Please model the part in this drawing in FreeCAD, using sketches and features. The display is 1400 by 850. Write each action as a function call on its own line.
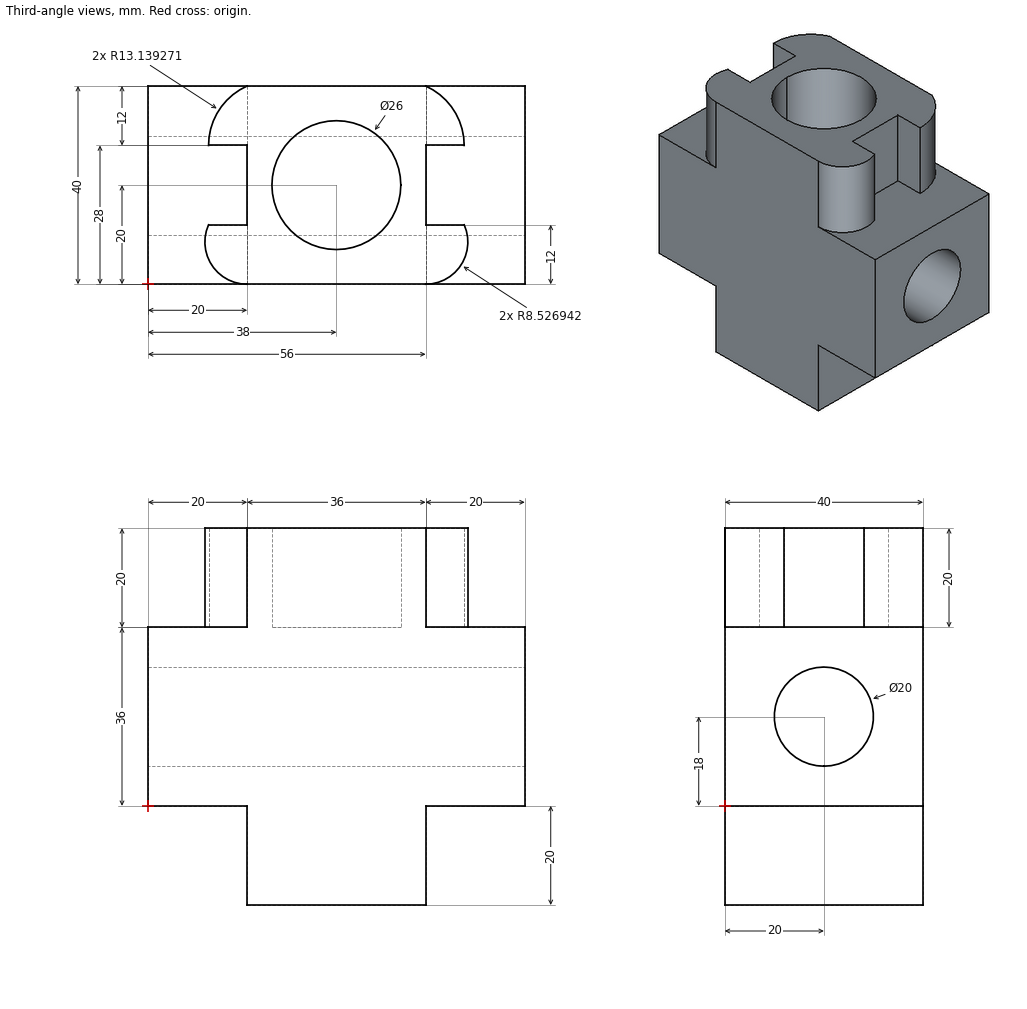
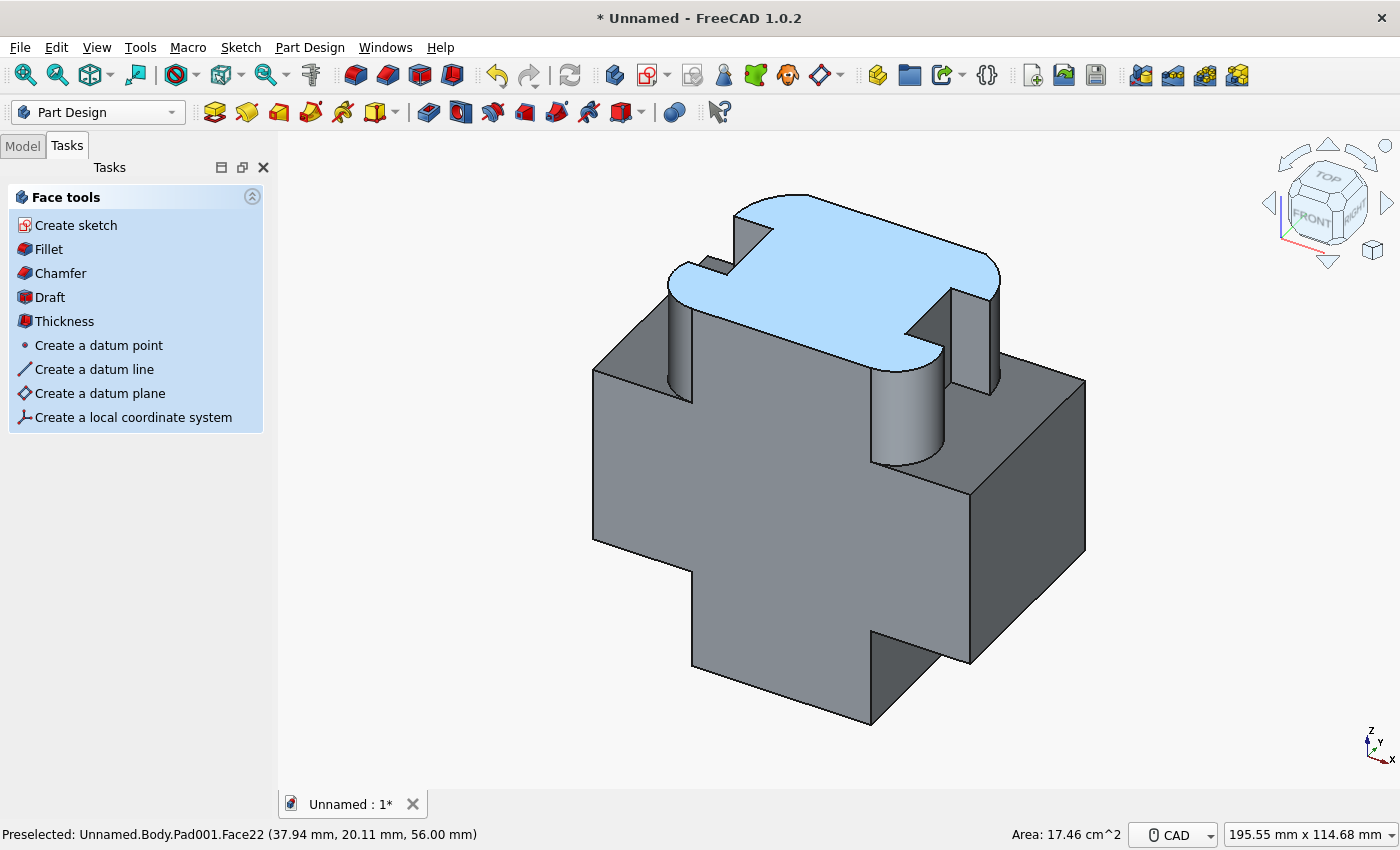
click(648, 76)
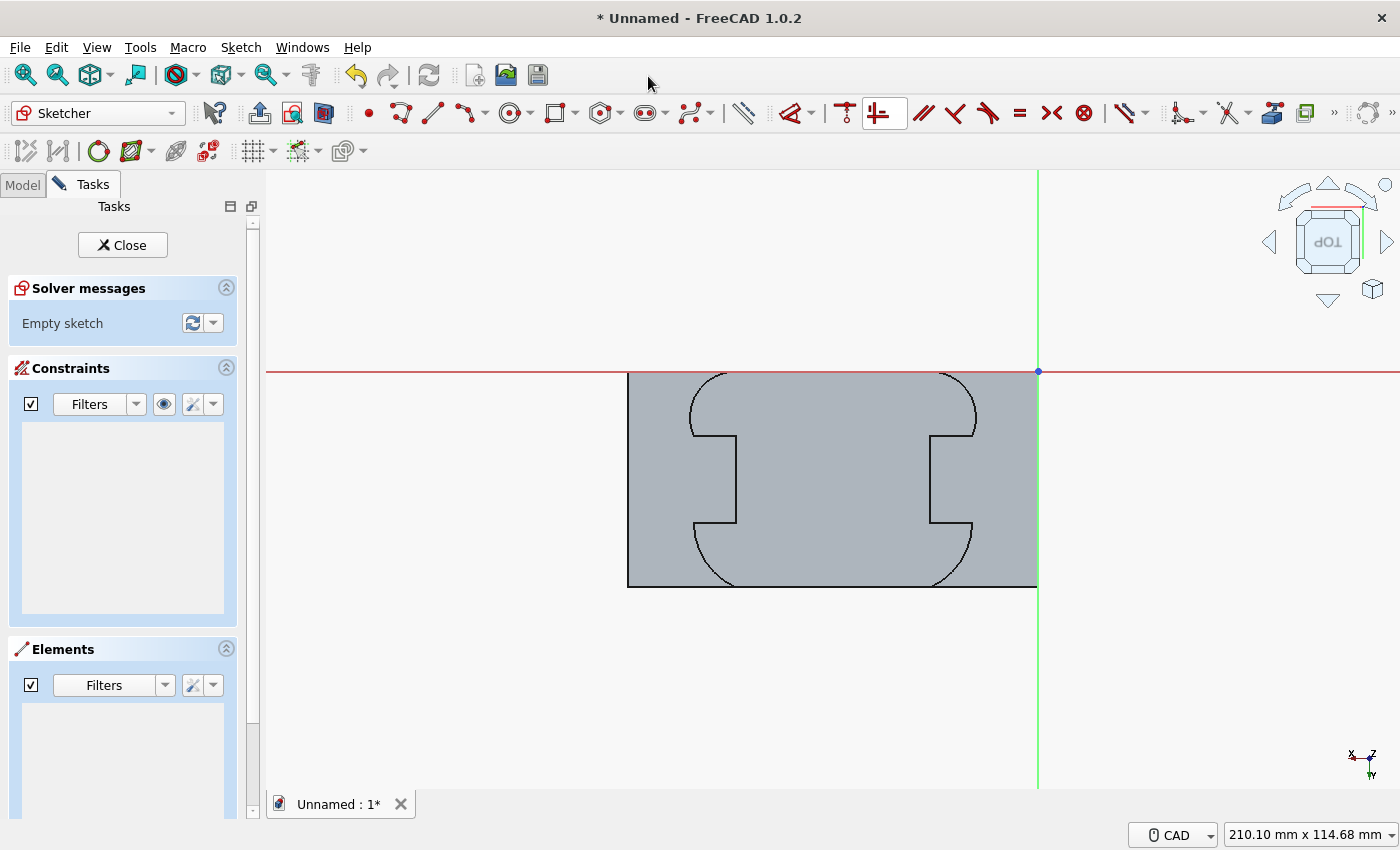
scroll(1011, 445, up, 4)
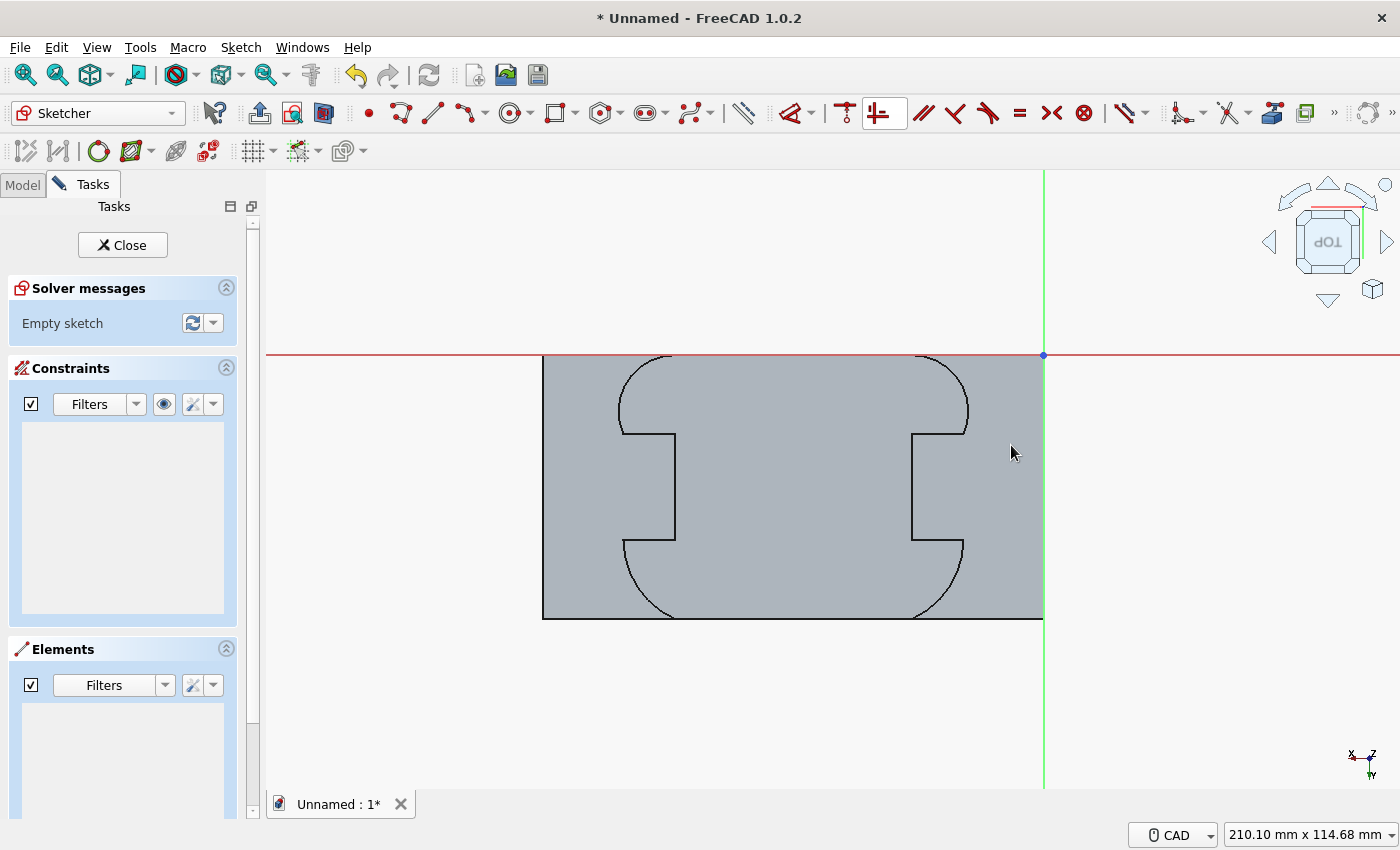
click(510, 114)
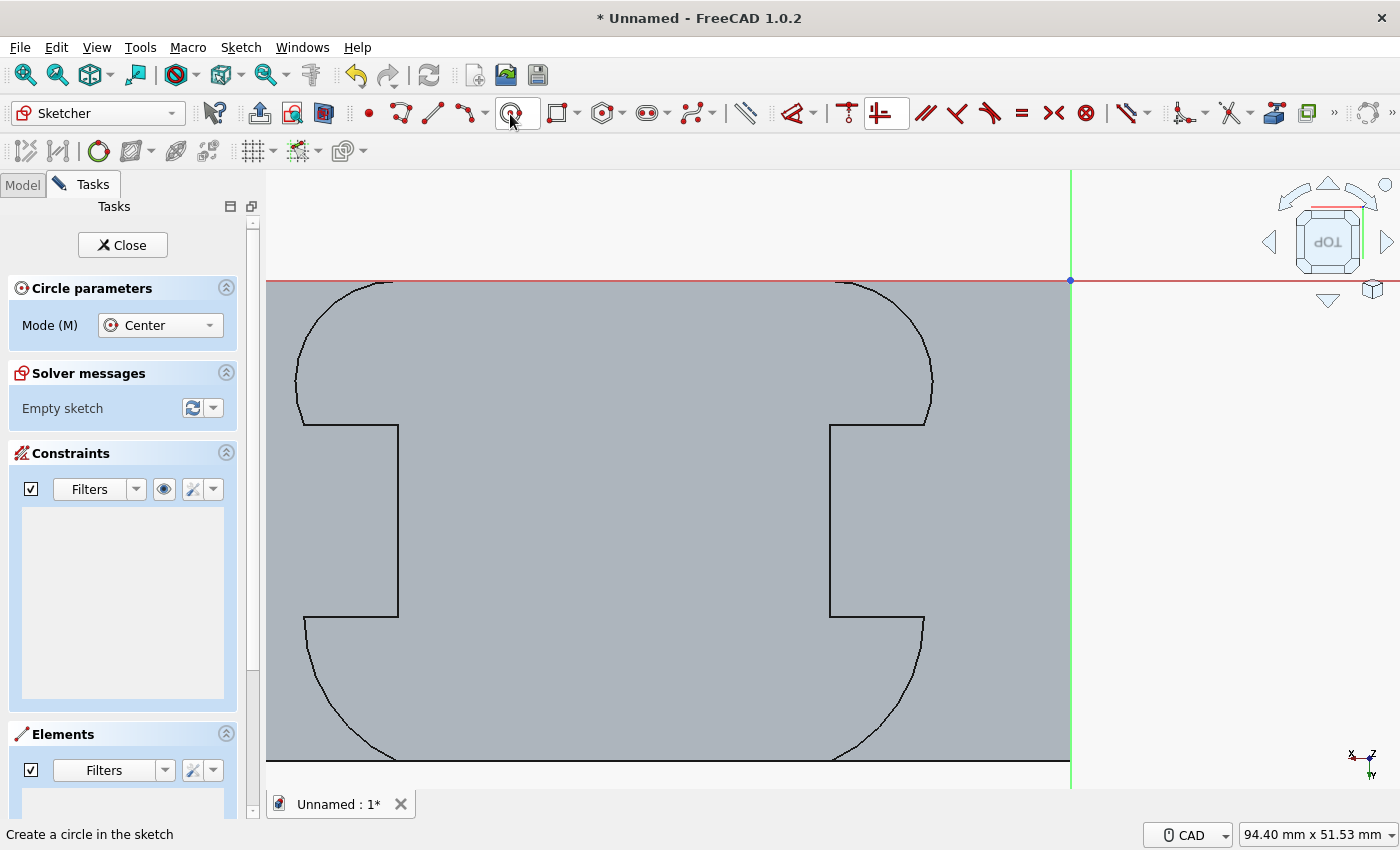
click(614, 521)
move(724, 411)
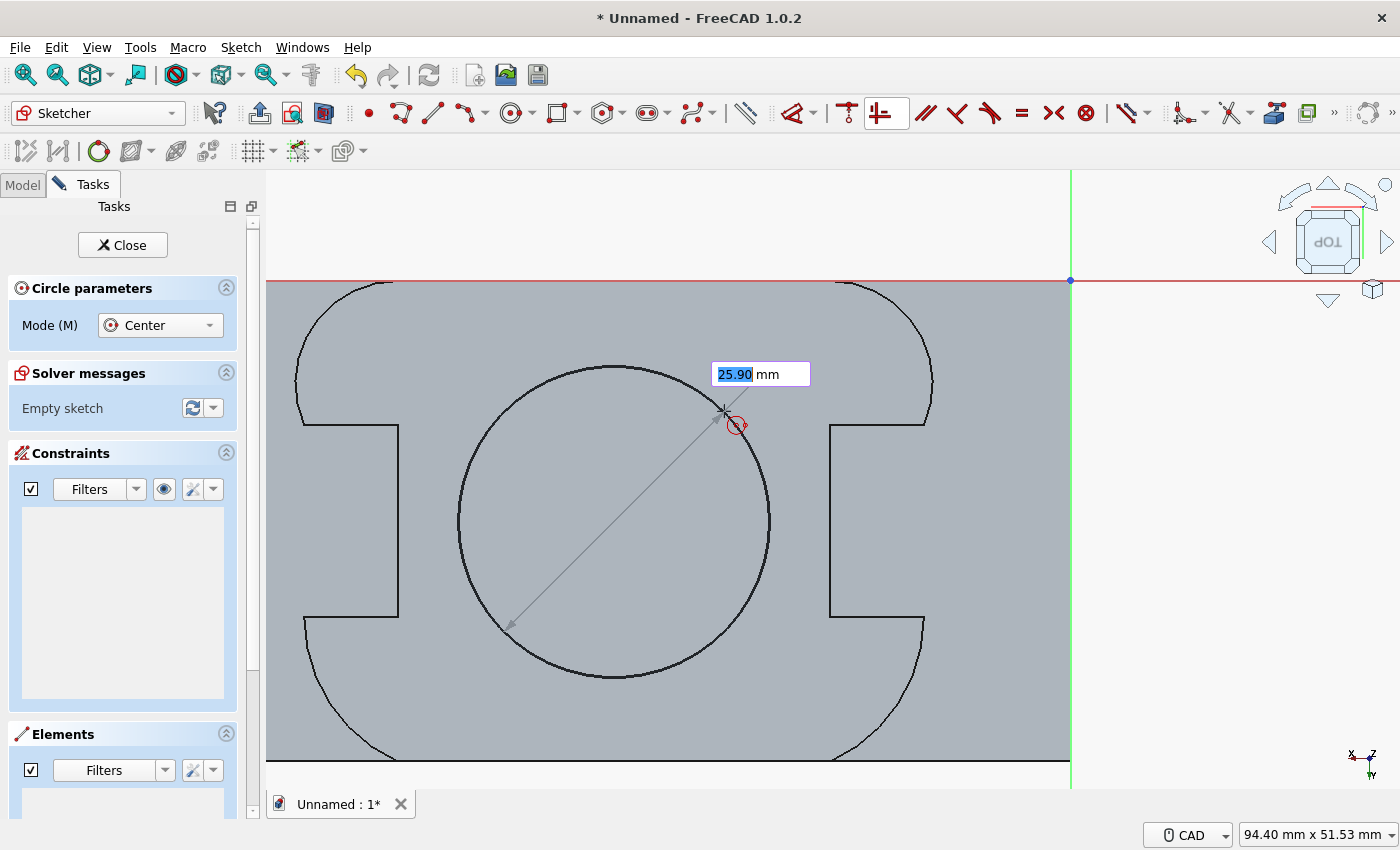
text(26)
key(Return)
key(Escape)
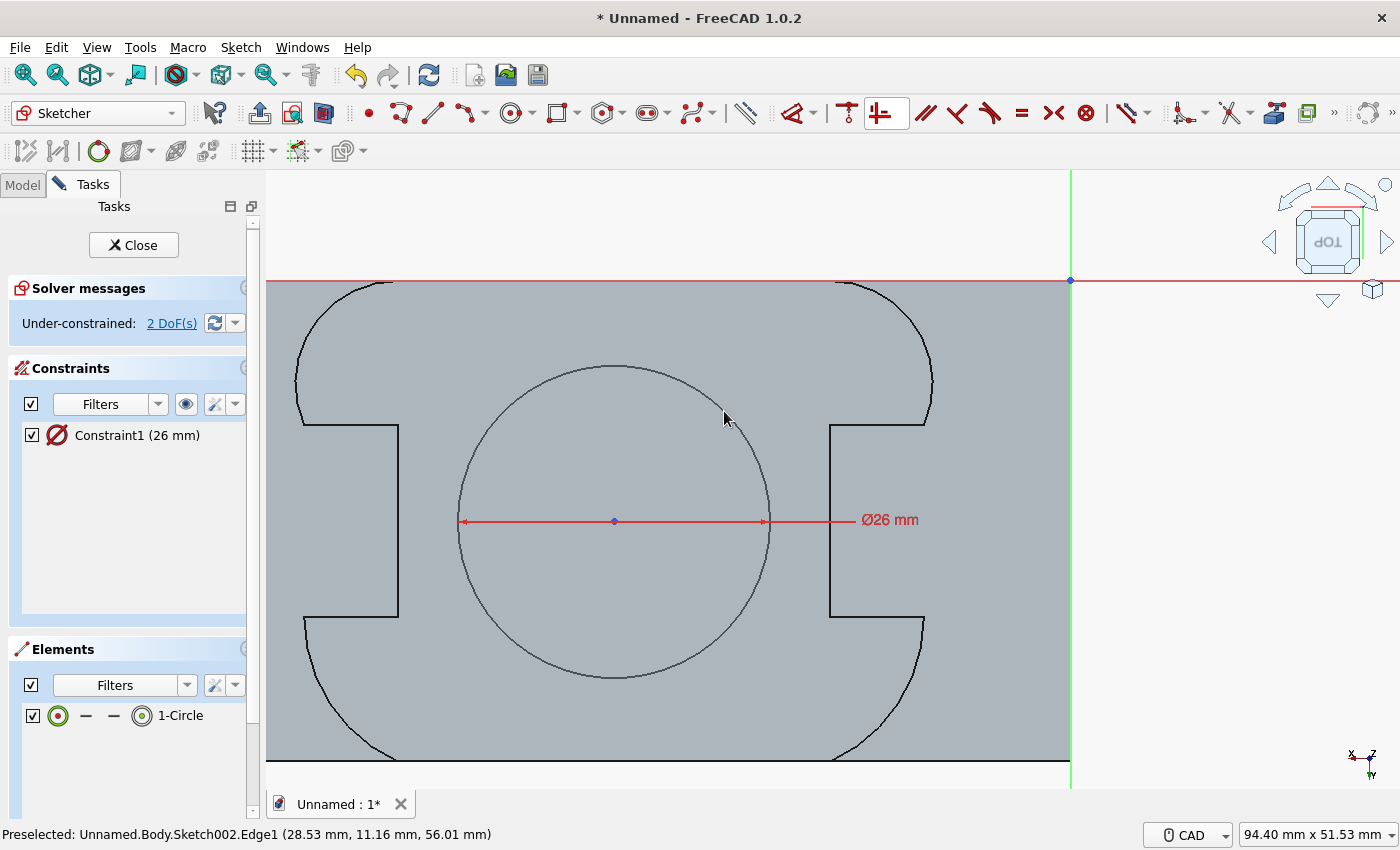
click(792, 114)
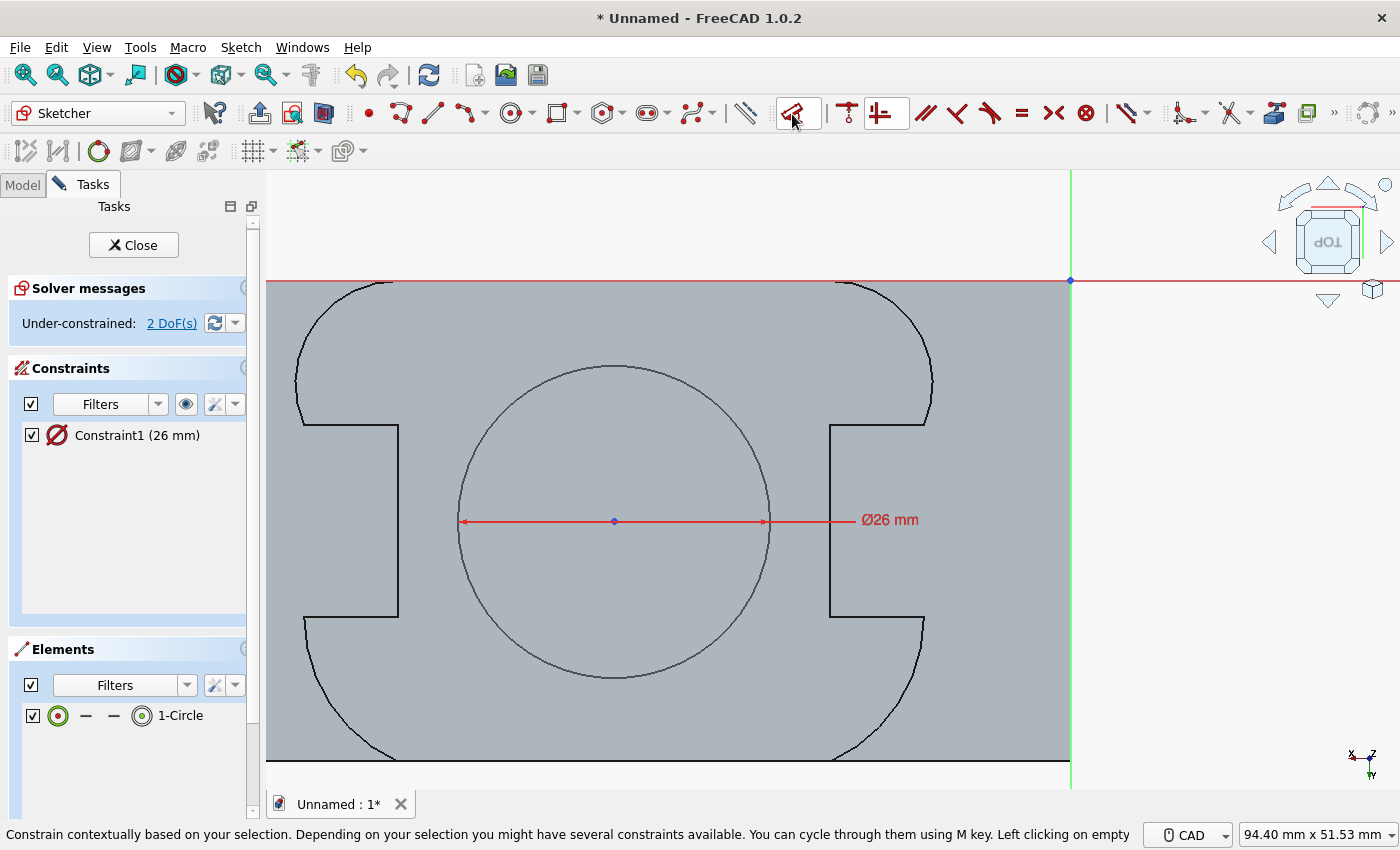
click(614, 522)
click(842, 247)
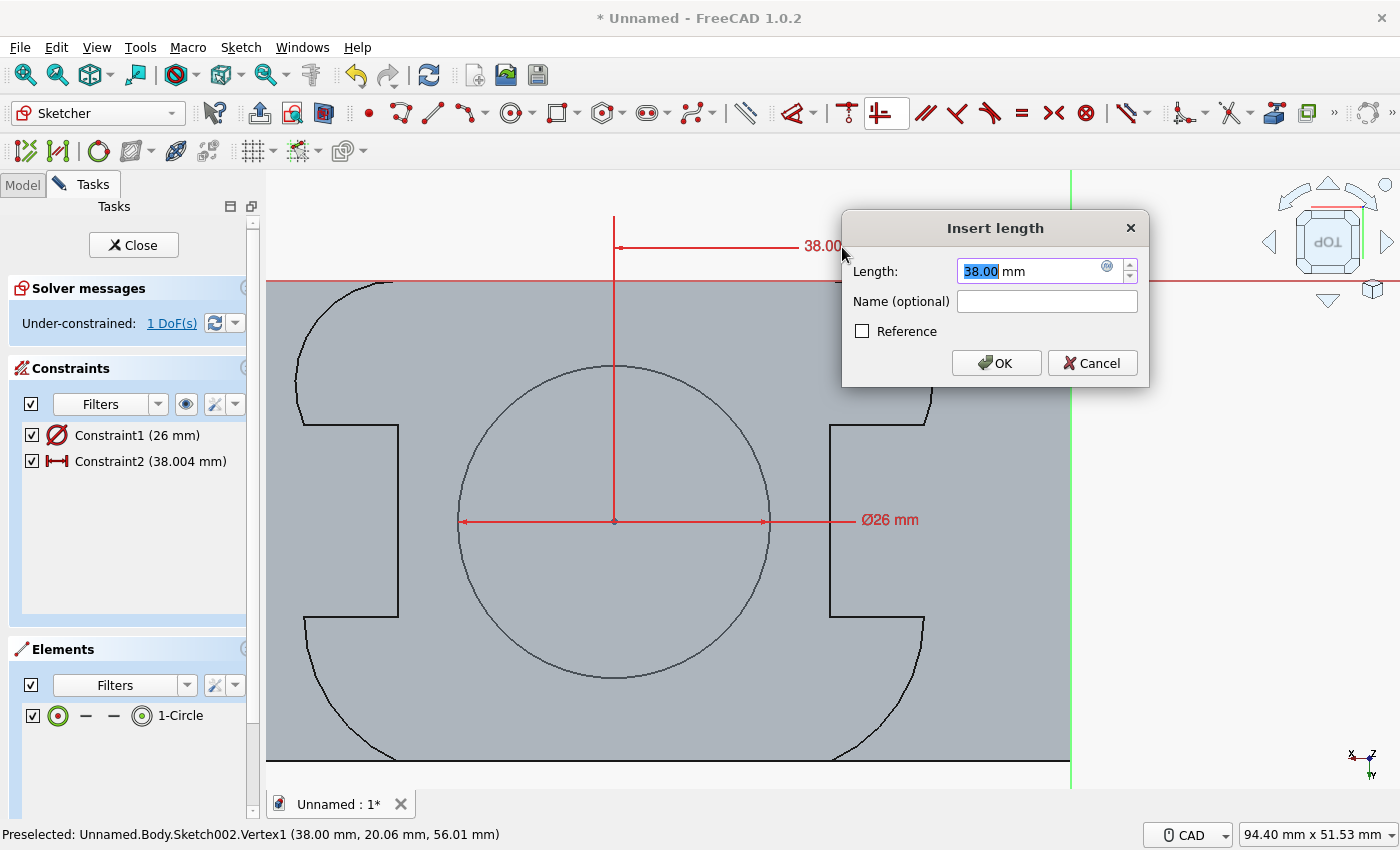
text(38)
key(Return)